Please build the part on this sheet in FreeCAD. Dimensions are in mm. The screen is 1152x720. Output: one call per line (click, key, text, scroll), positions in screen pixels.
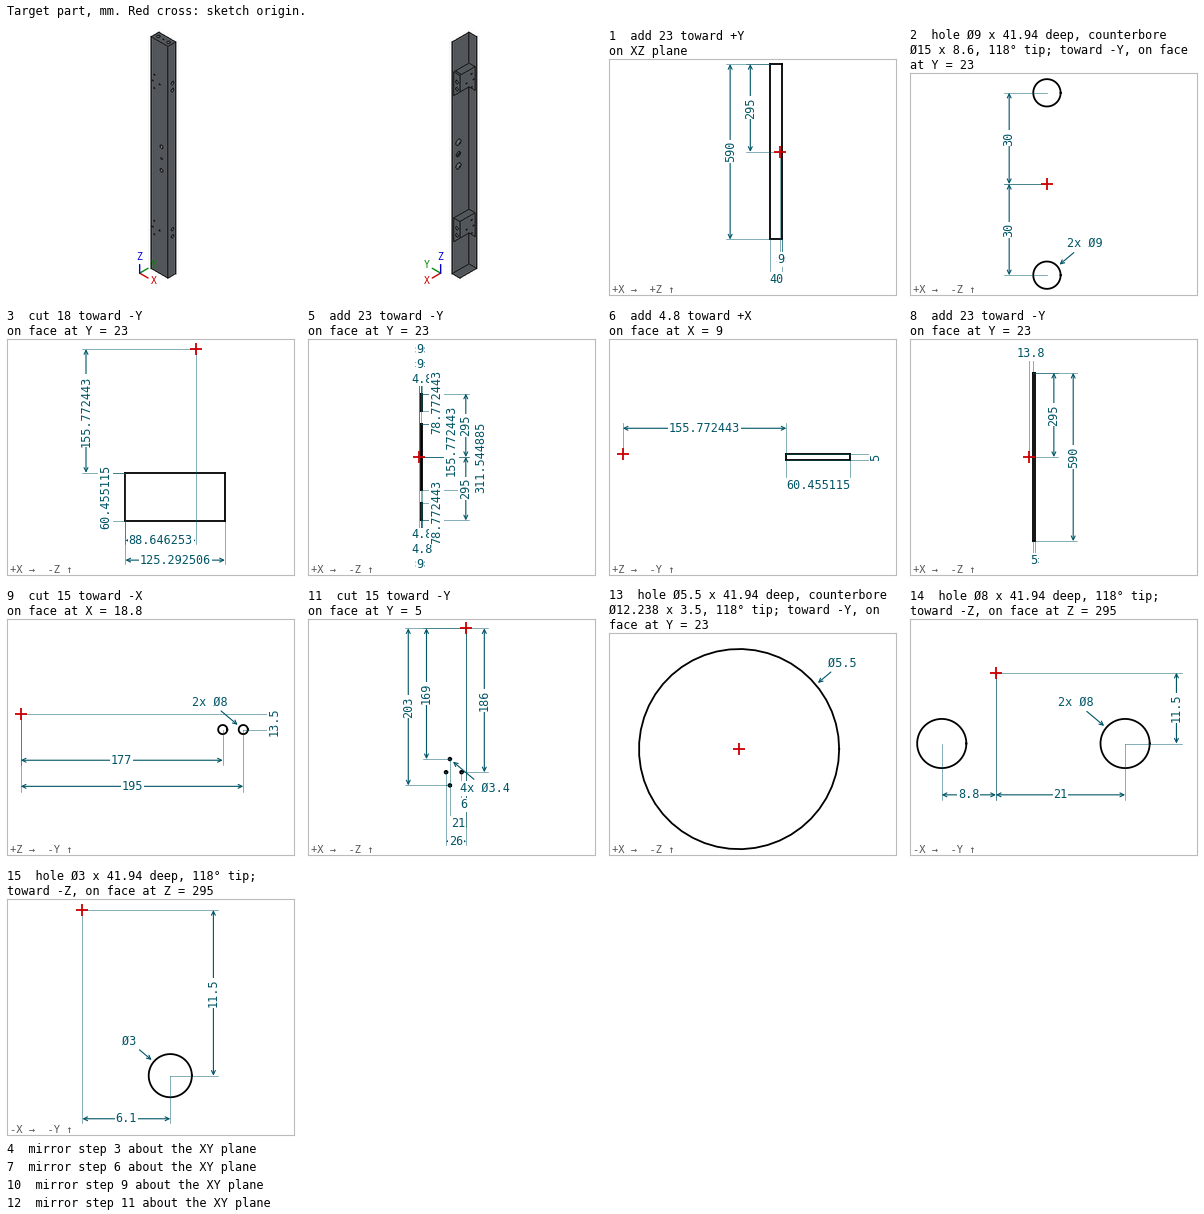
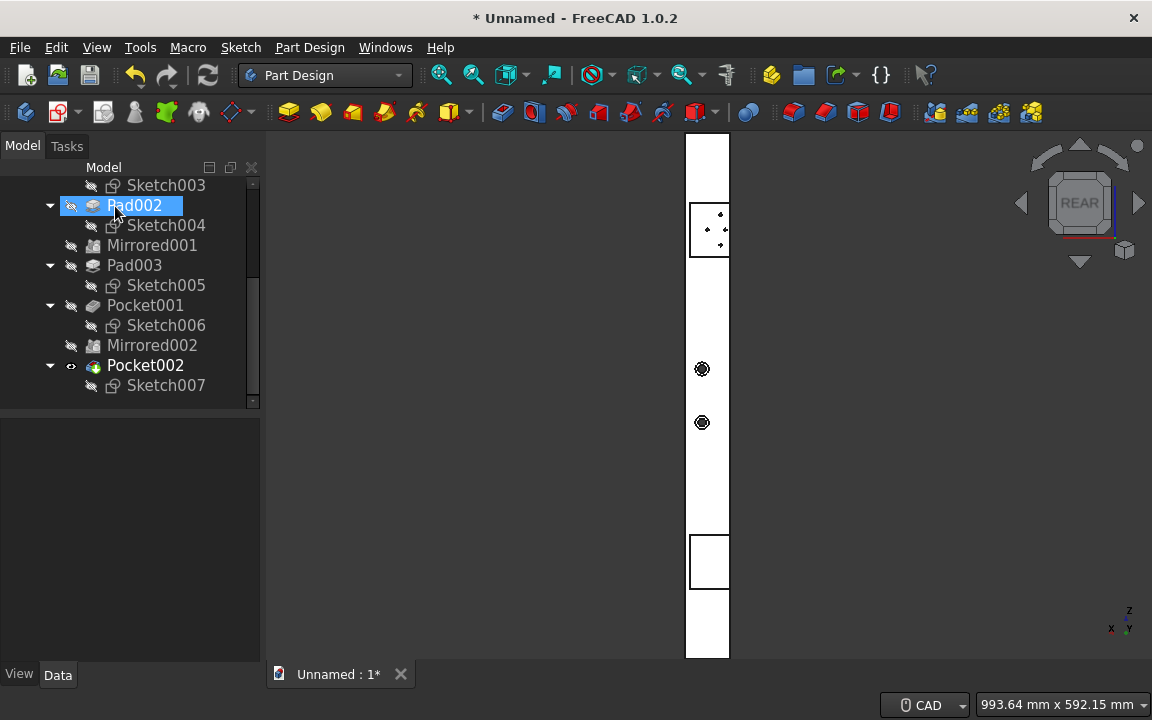
click(116, 366)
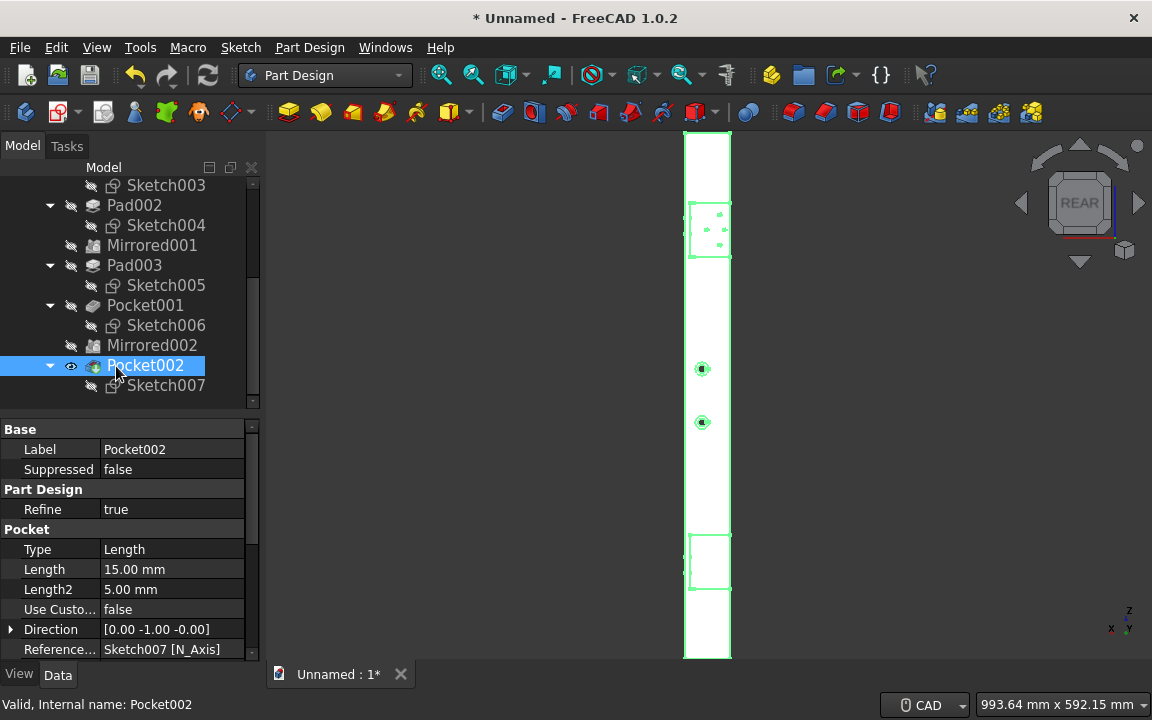
click(936, 112)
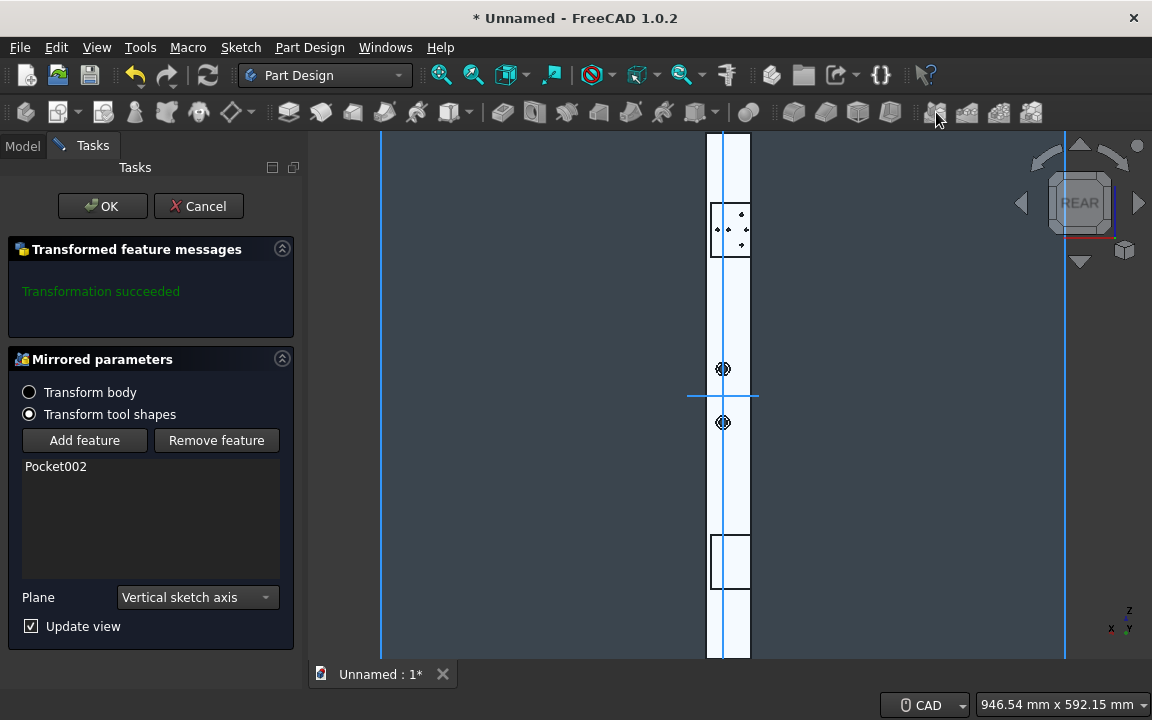
click(198, 598)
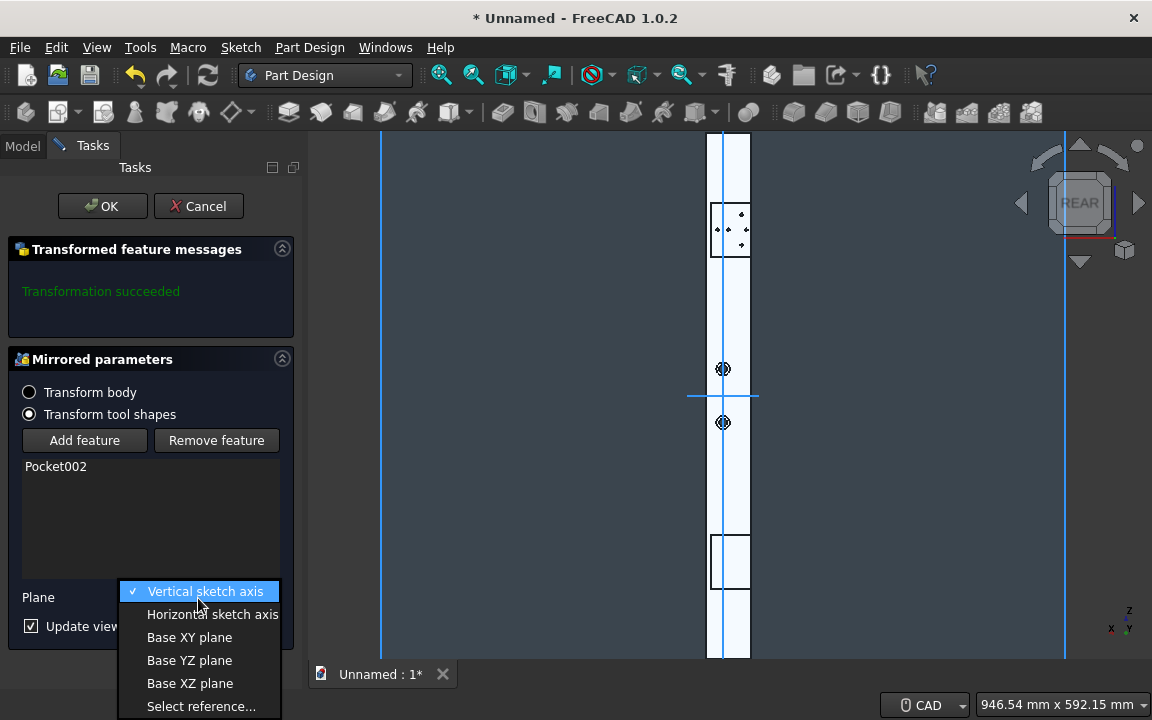
click(198, 638)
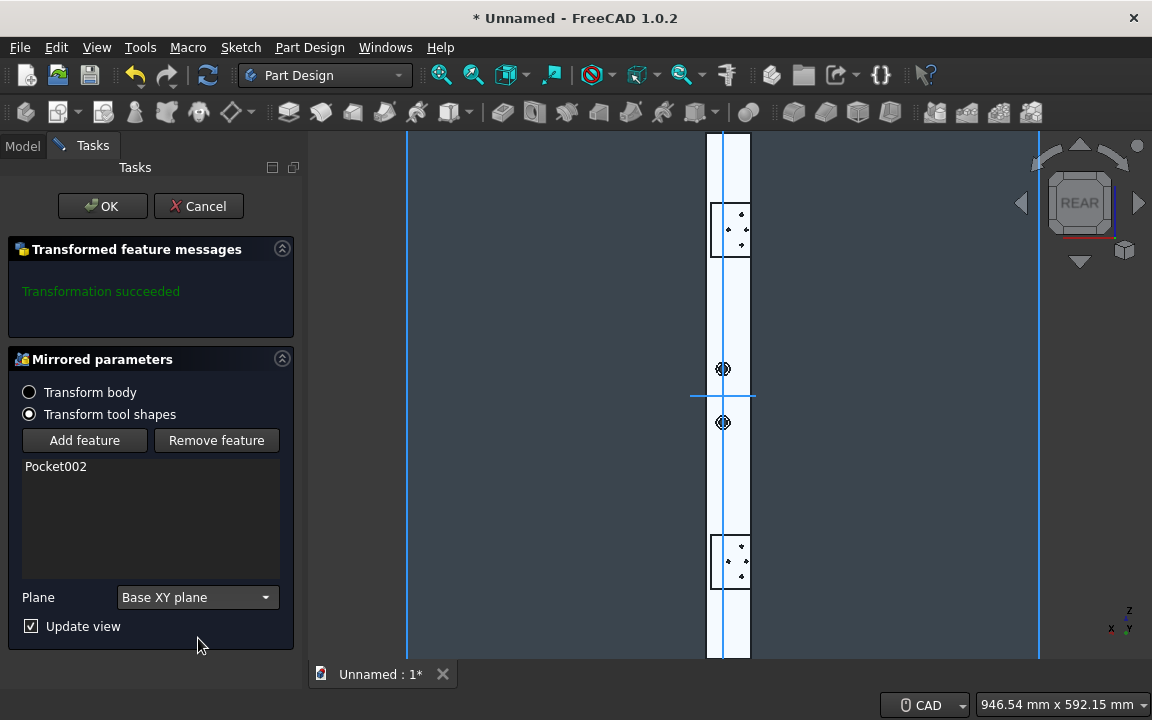
click(103, 206)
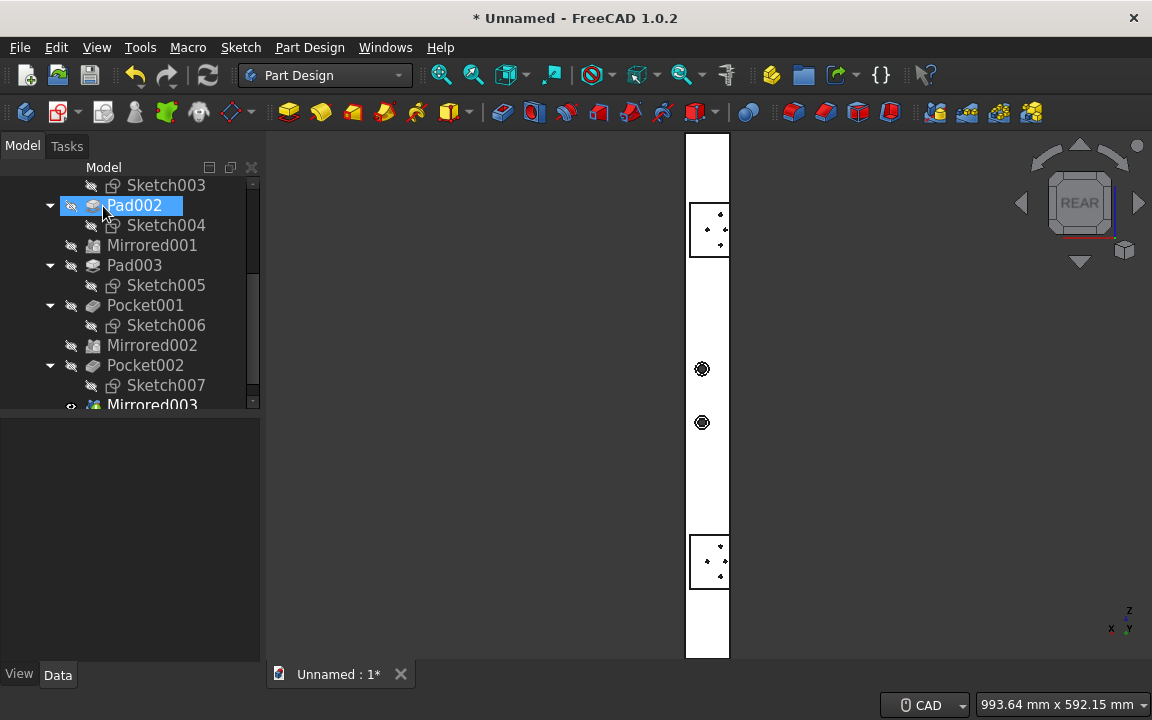
click(707, 620)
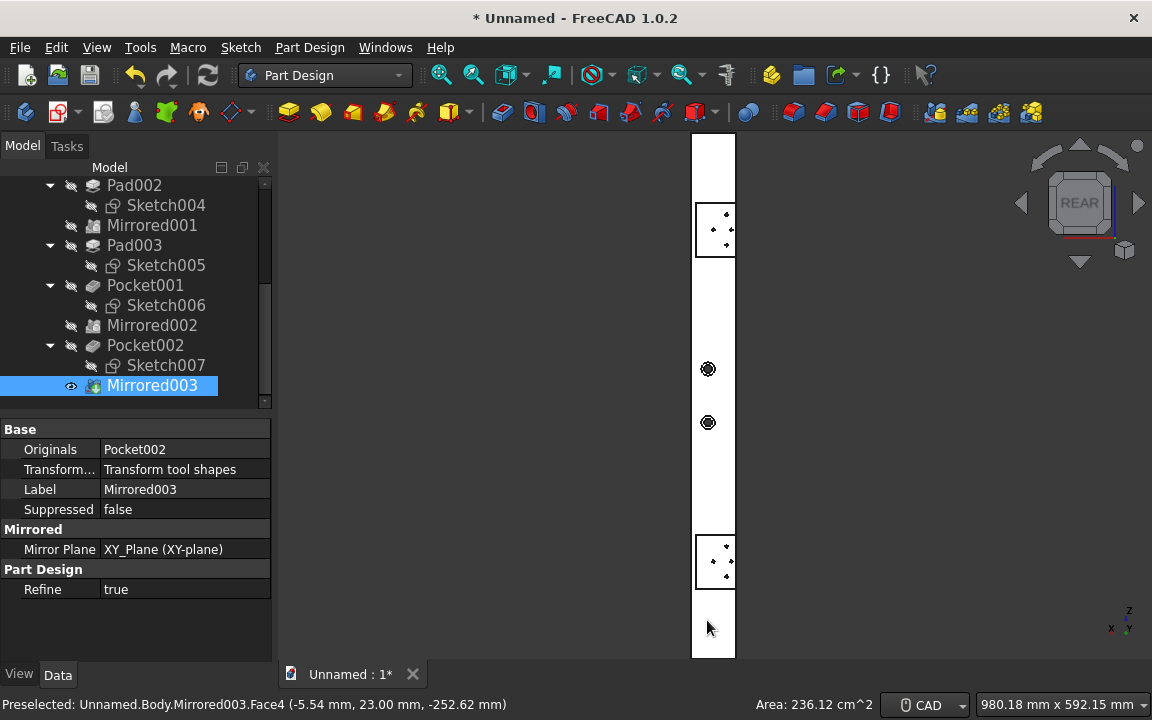
click(58, 112)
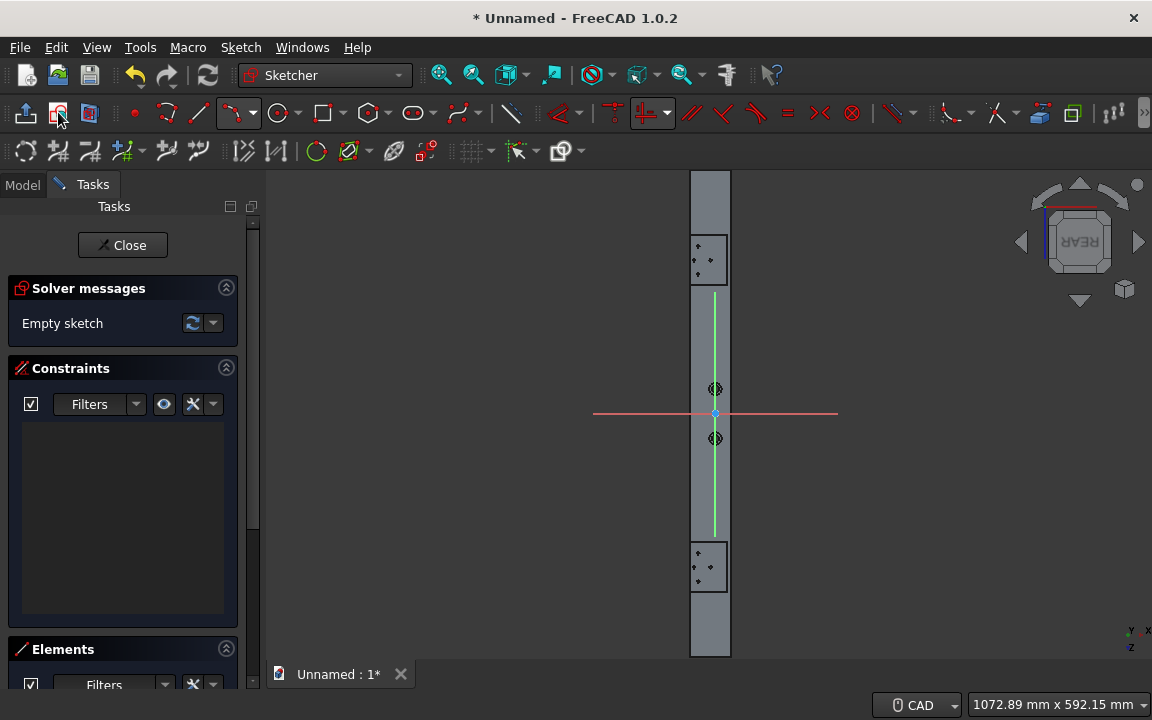
scroll(719, 414, up, 15)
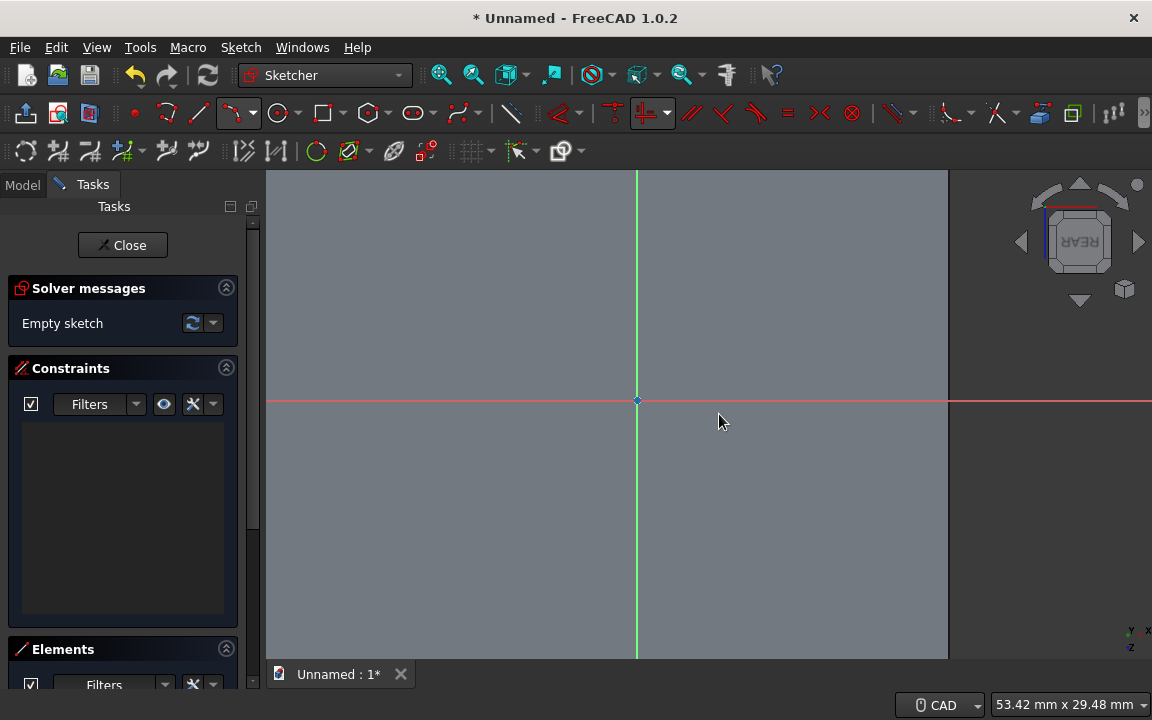
scroll(636, 395, up, 6)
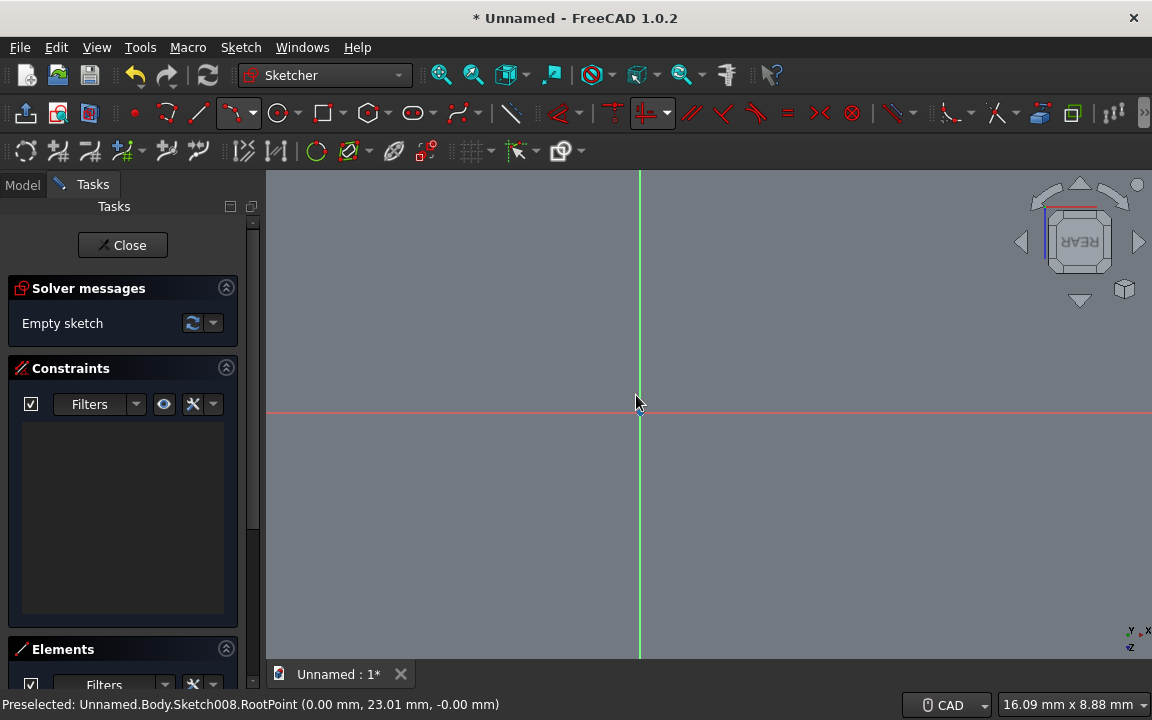
click(278, 114)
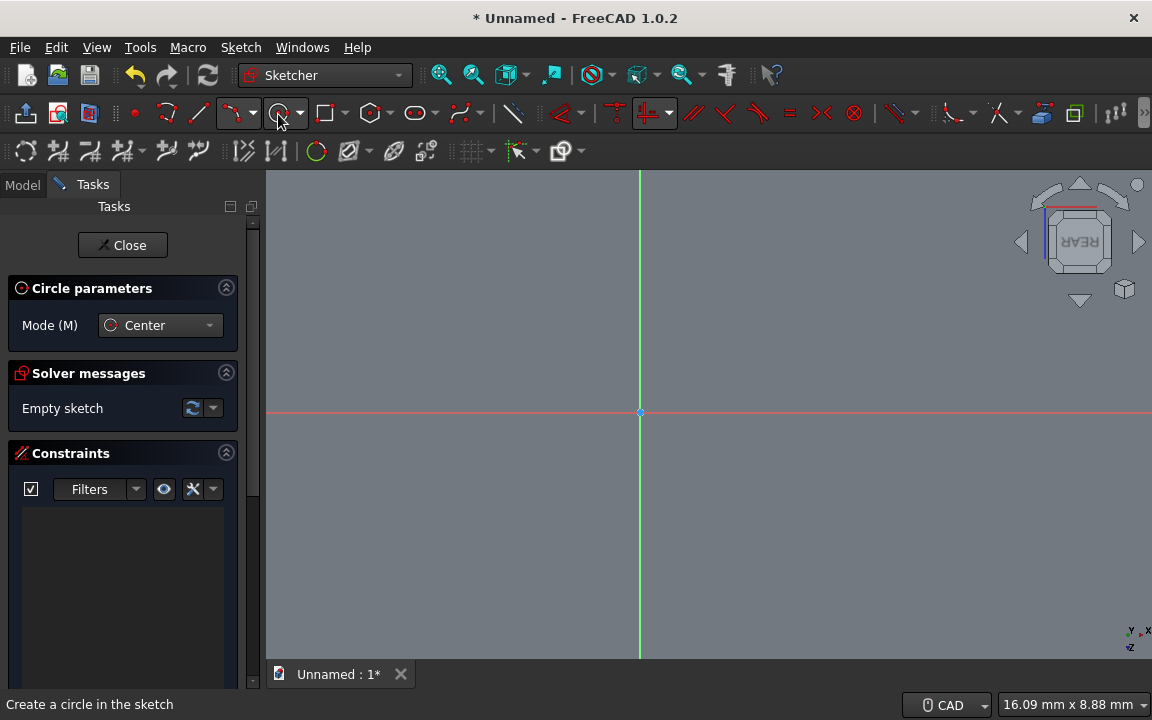
click(640, 413)
click(747, 306)
key(Escape)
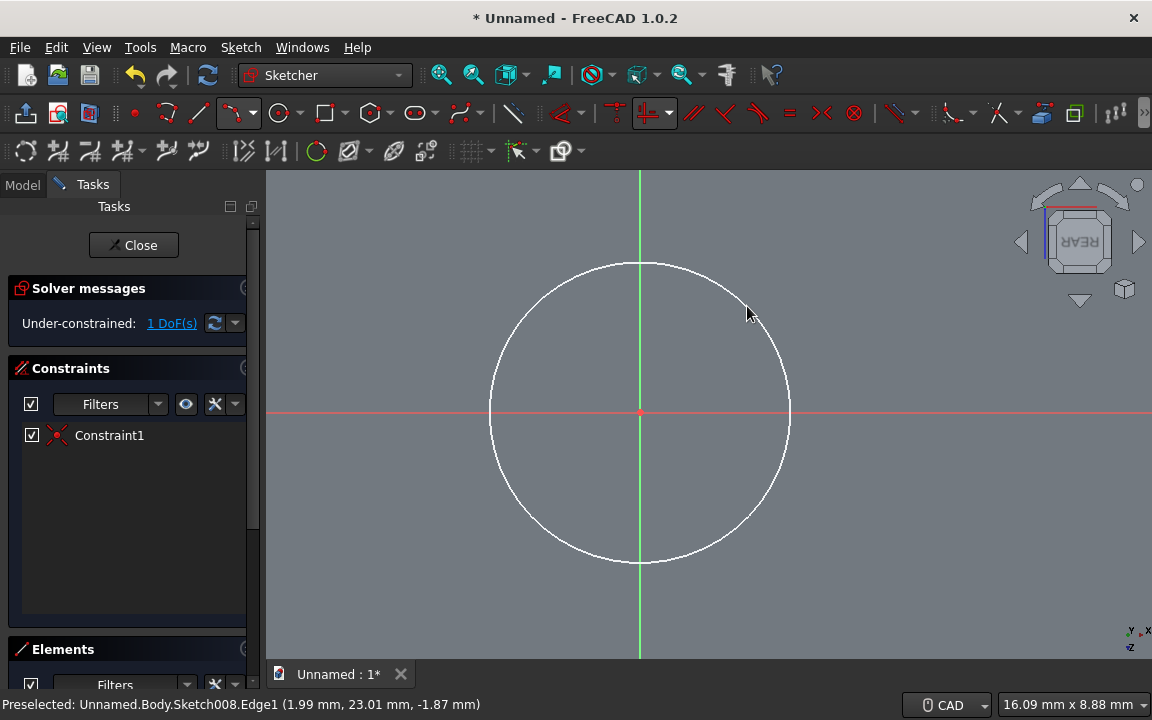
click(560, 114)